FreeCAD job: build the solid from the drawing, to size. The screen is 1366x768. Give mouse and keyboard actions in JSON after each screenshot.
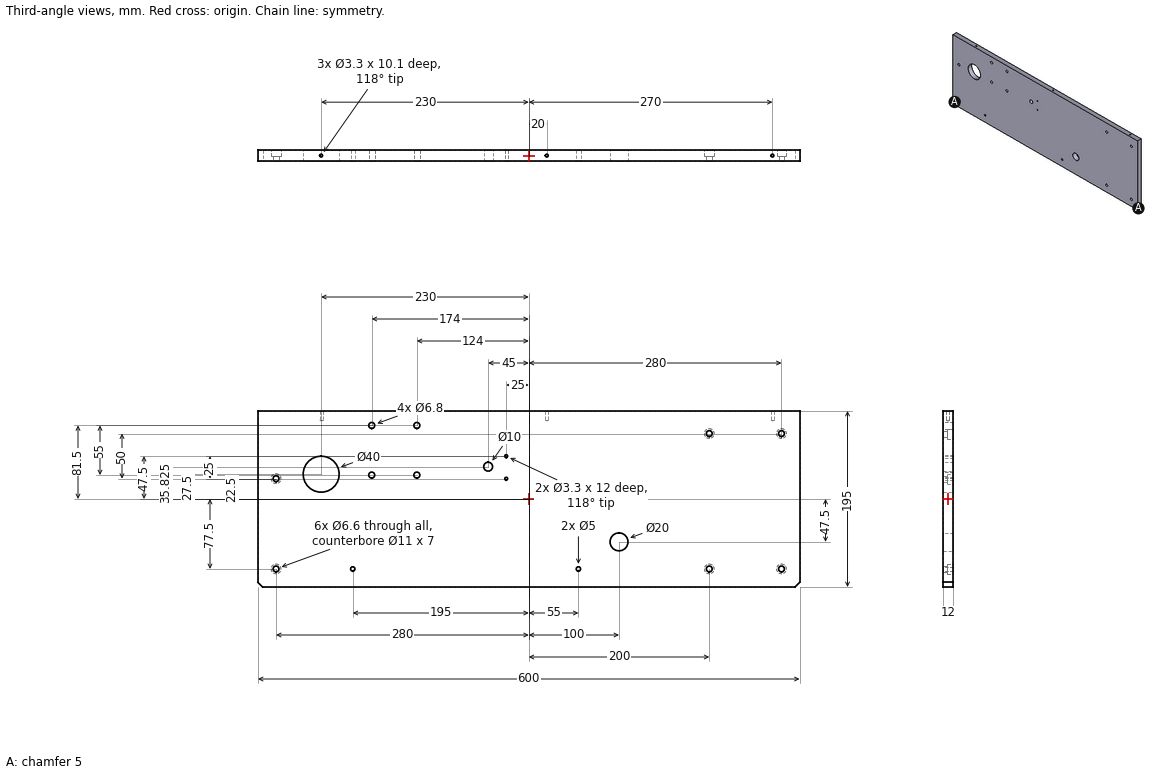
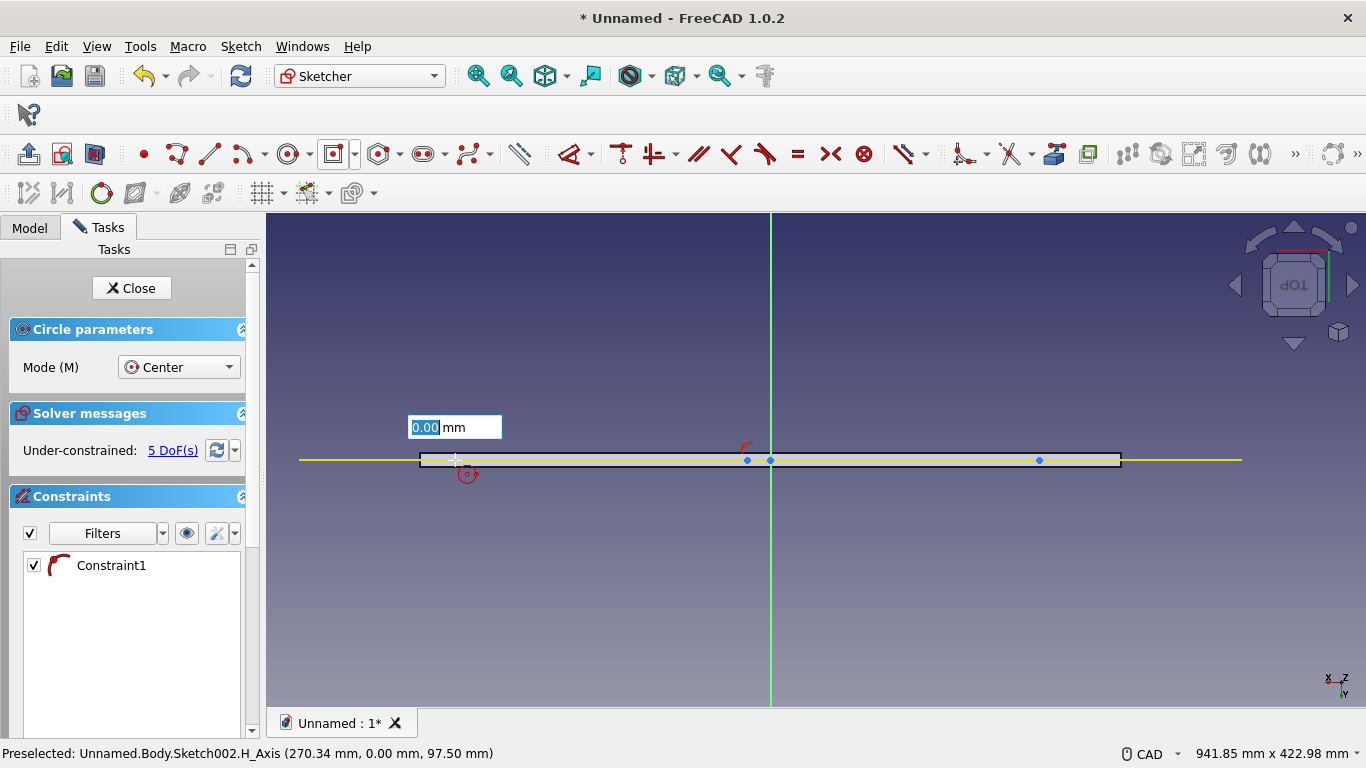
{"action": "scroll", "coordinate": [455, 462], "scroll_direction": "up", "scroll_amount": 11}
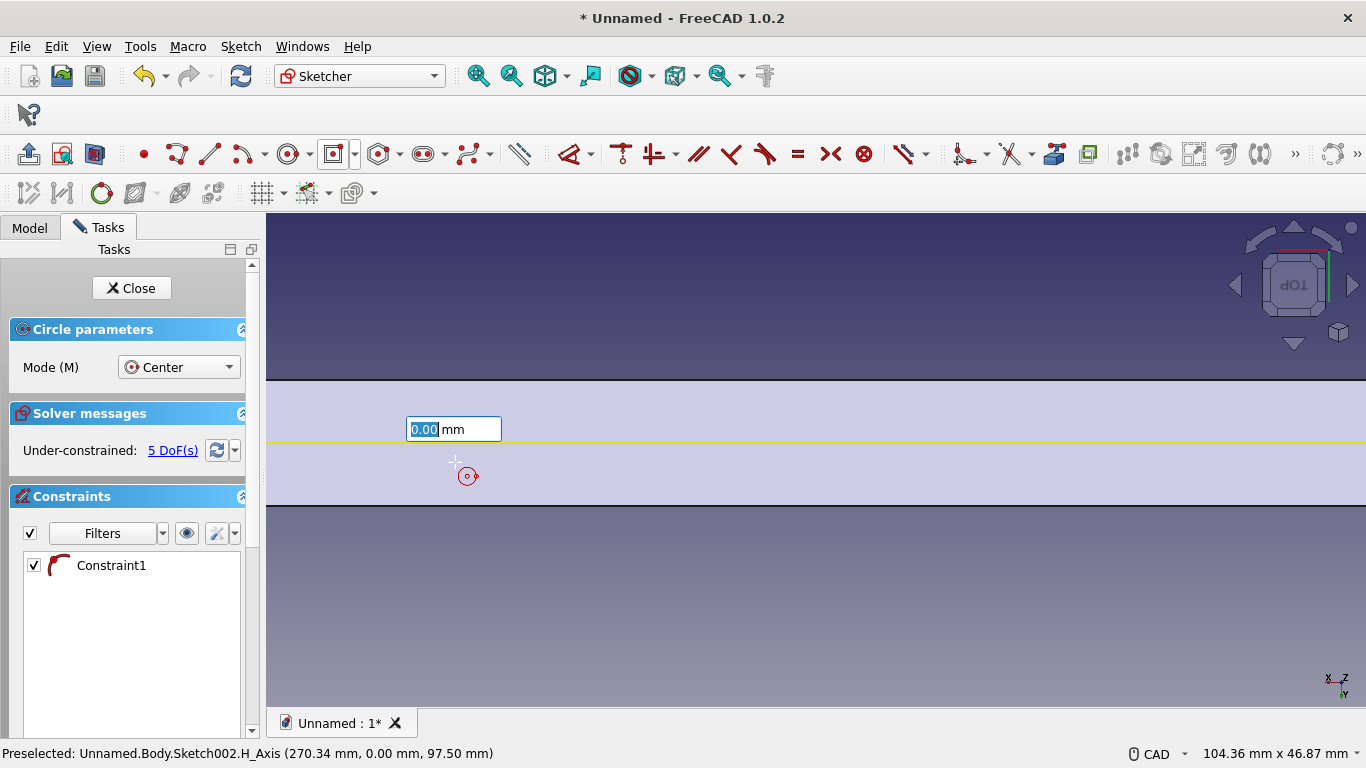
{"action": "left_click", "coordinate": [451, 459]}
{"action": "key", "text": "Escape"}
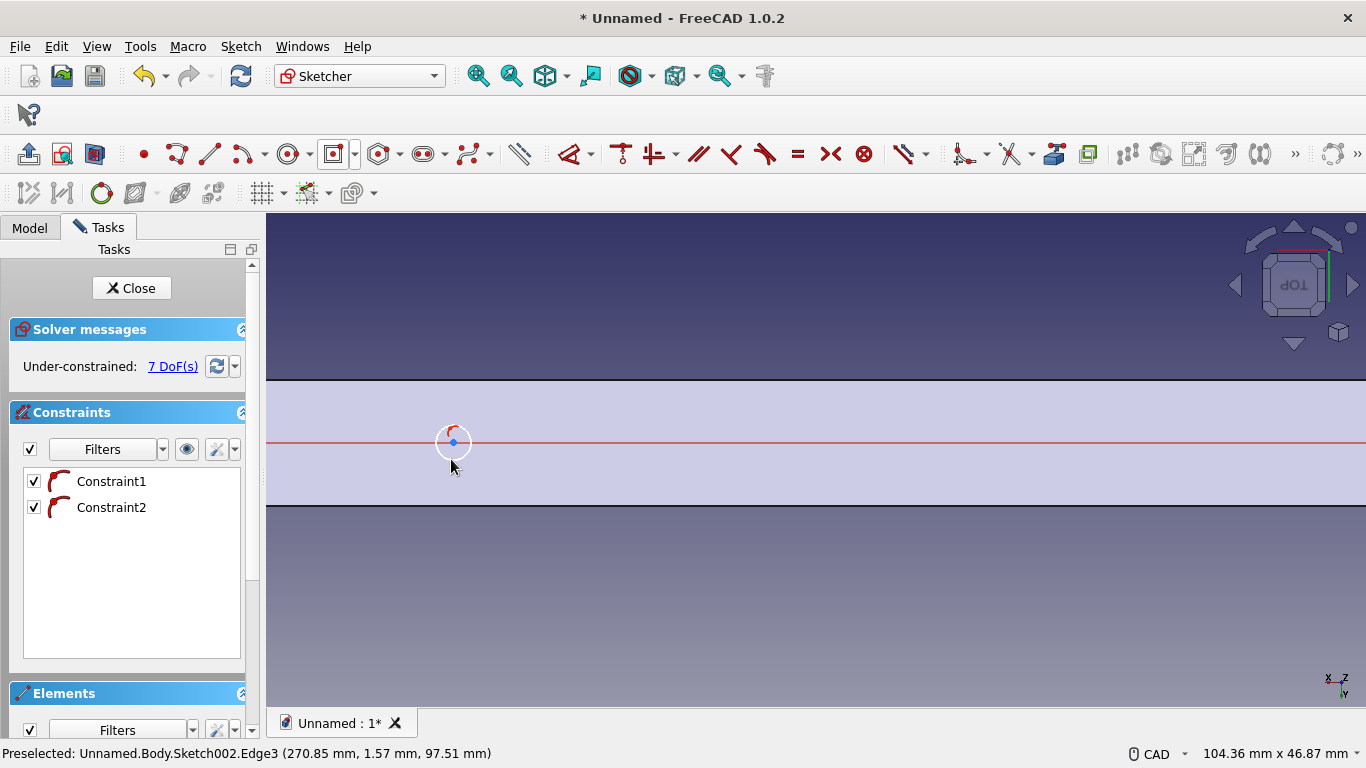
{"action": "scroll", "coordinate": [455, 462], "scroll_direction": "down", "scroll_amount": 11}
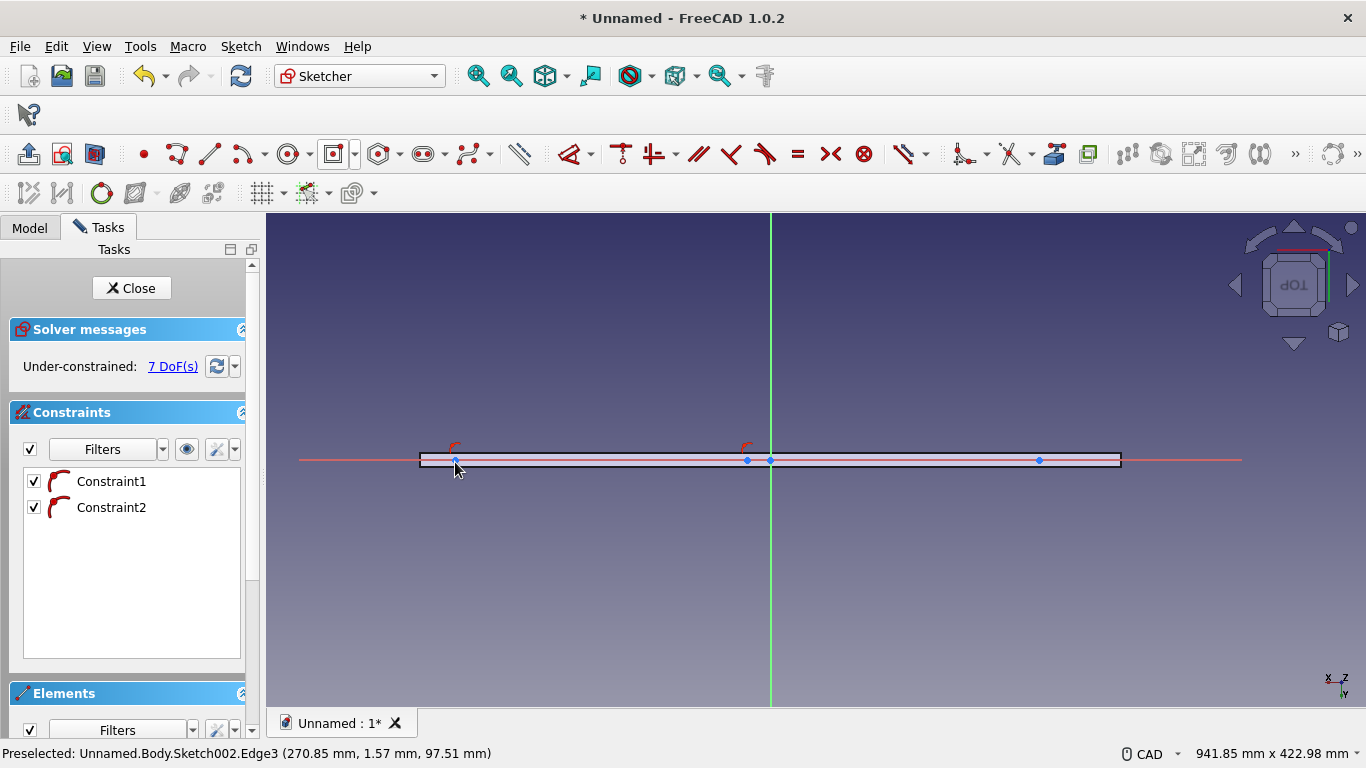
{"action": "scroll", "coordinate": [1040, 460], "scroll_direction": "up", "scroll_amount": 12}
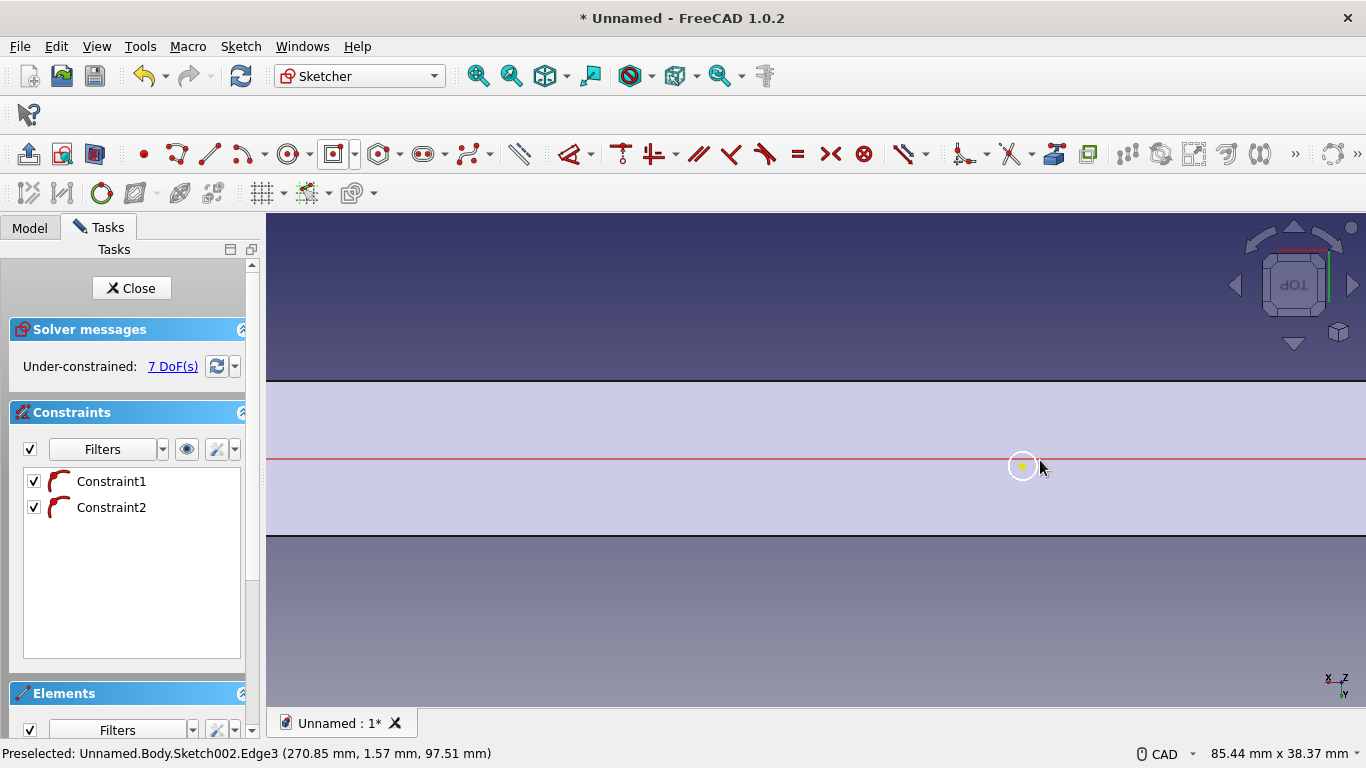
{"action": "left_click", "coordinate": [1033, 456]}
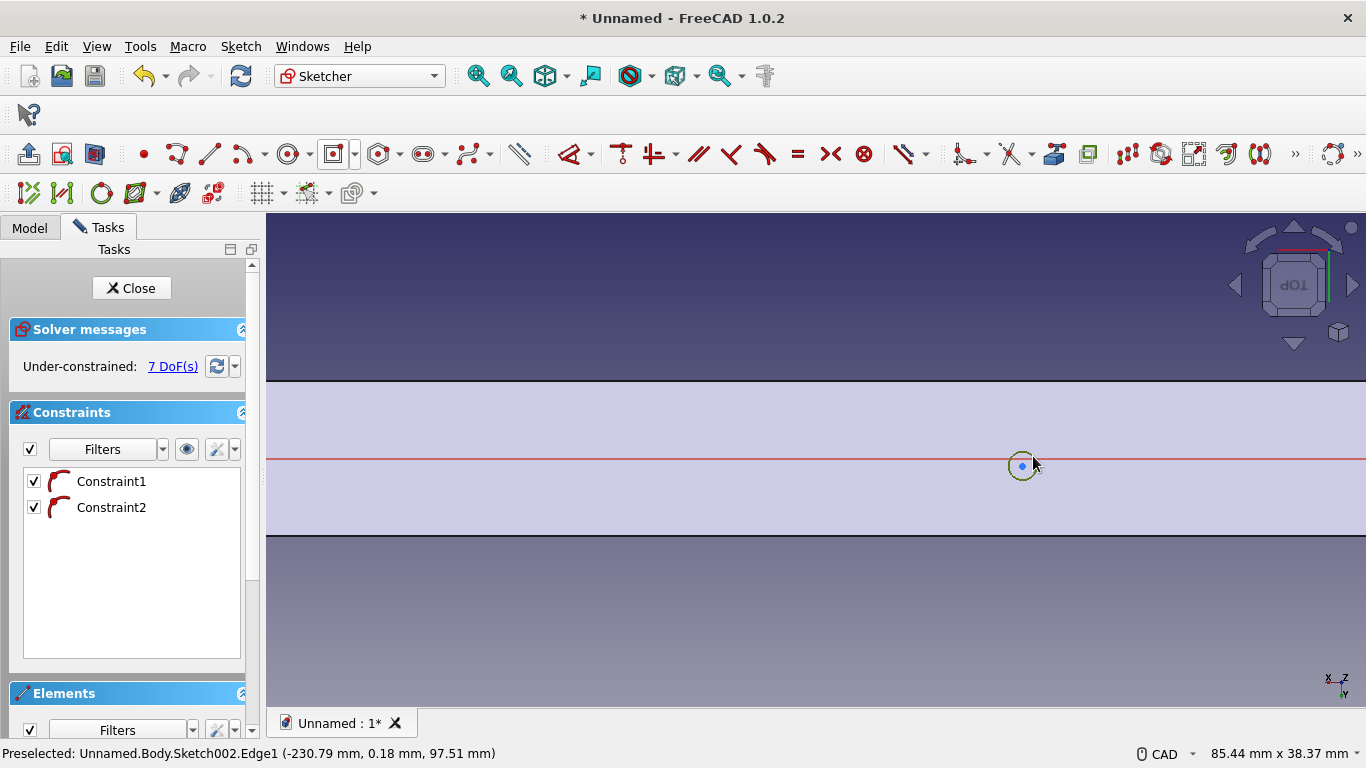
{"action": "scroll", "coordinate": [1041, 460], "scroll_direction": "down", "scroll_amount": 12}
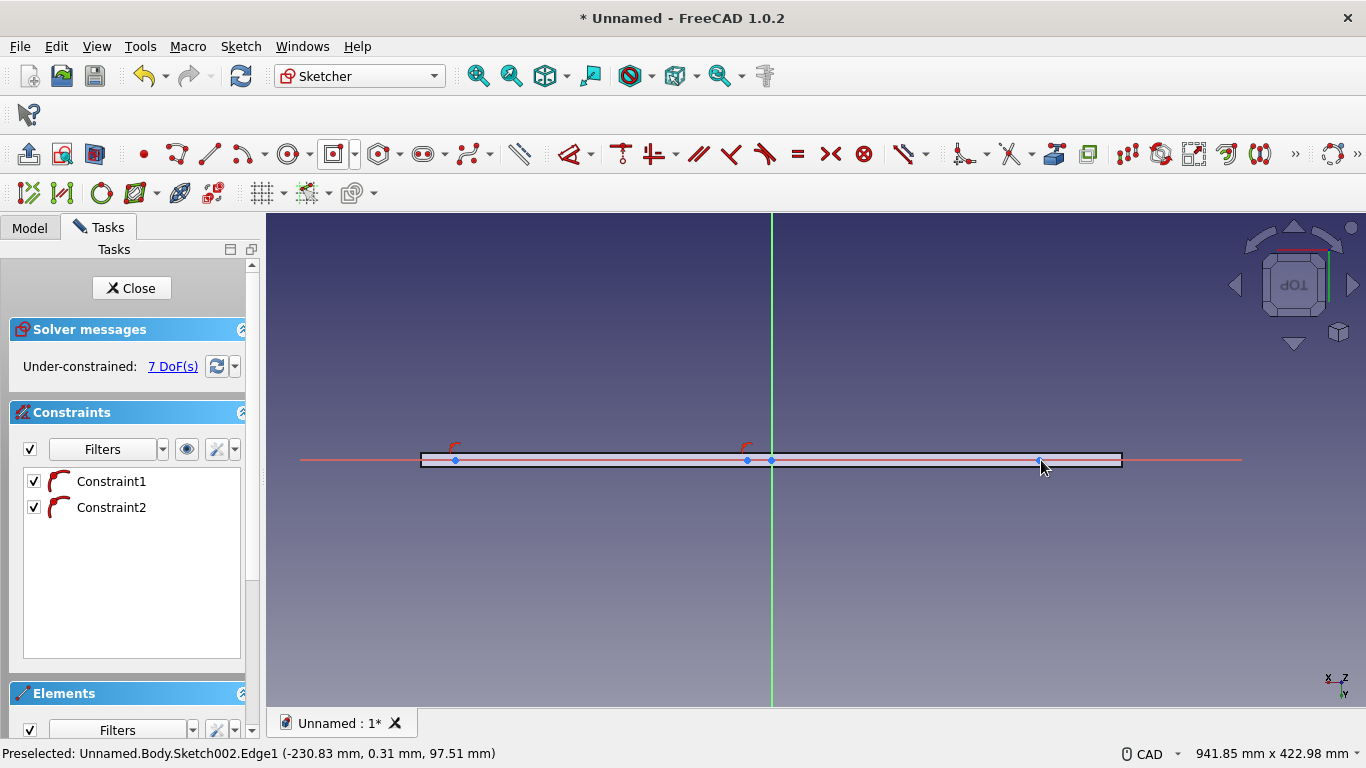
{"action": "scroll", "coordinate": [749, 459], "scroll_direction": "up", "scroll_amount": 12}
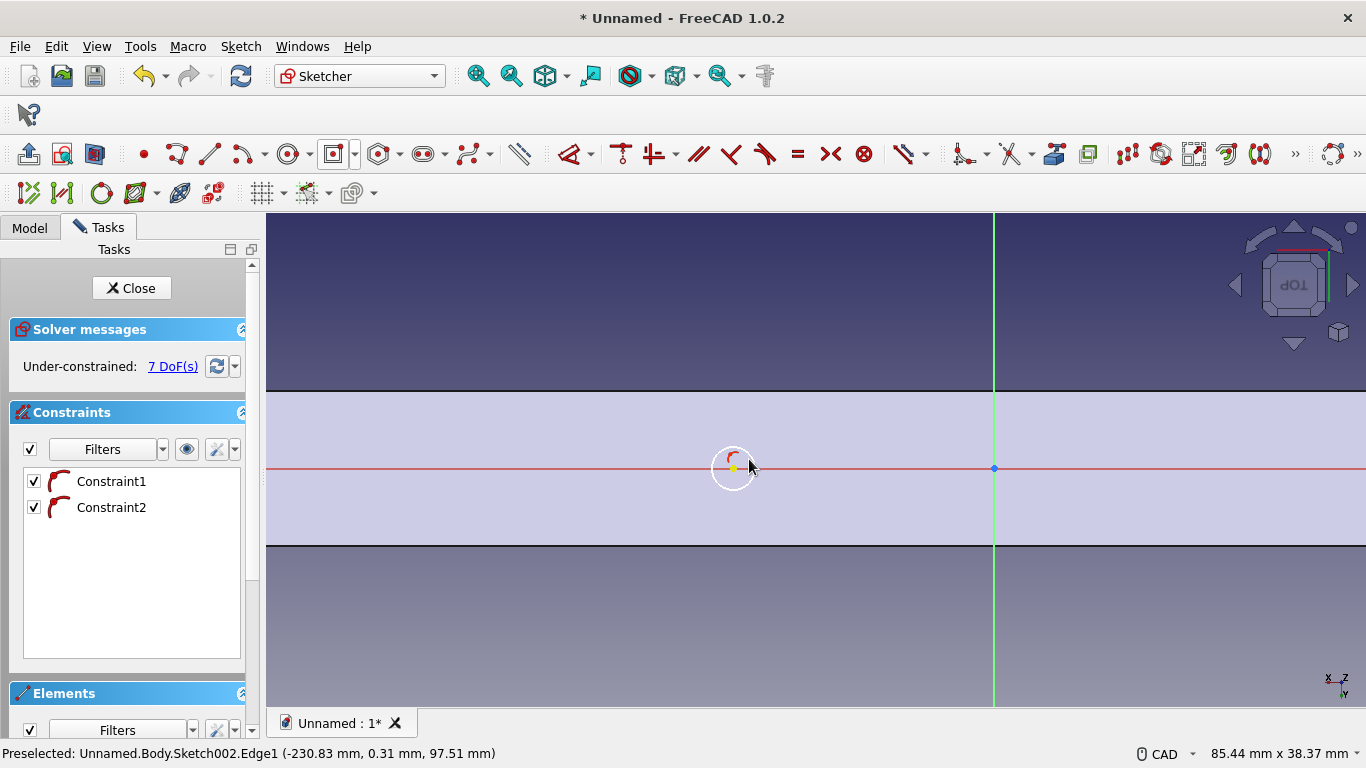
{"action": "left_click", "coordinate": [748, 453]}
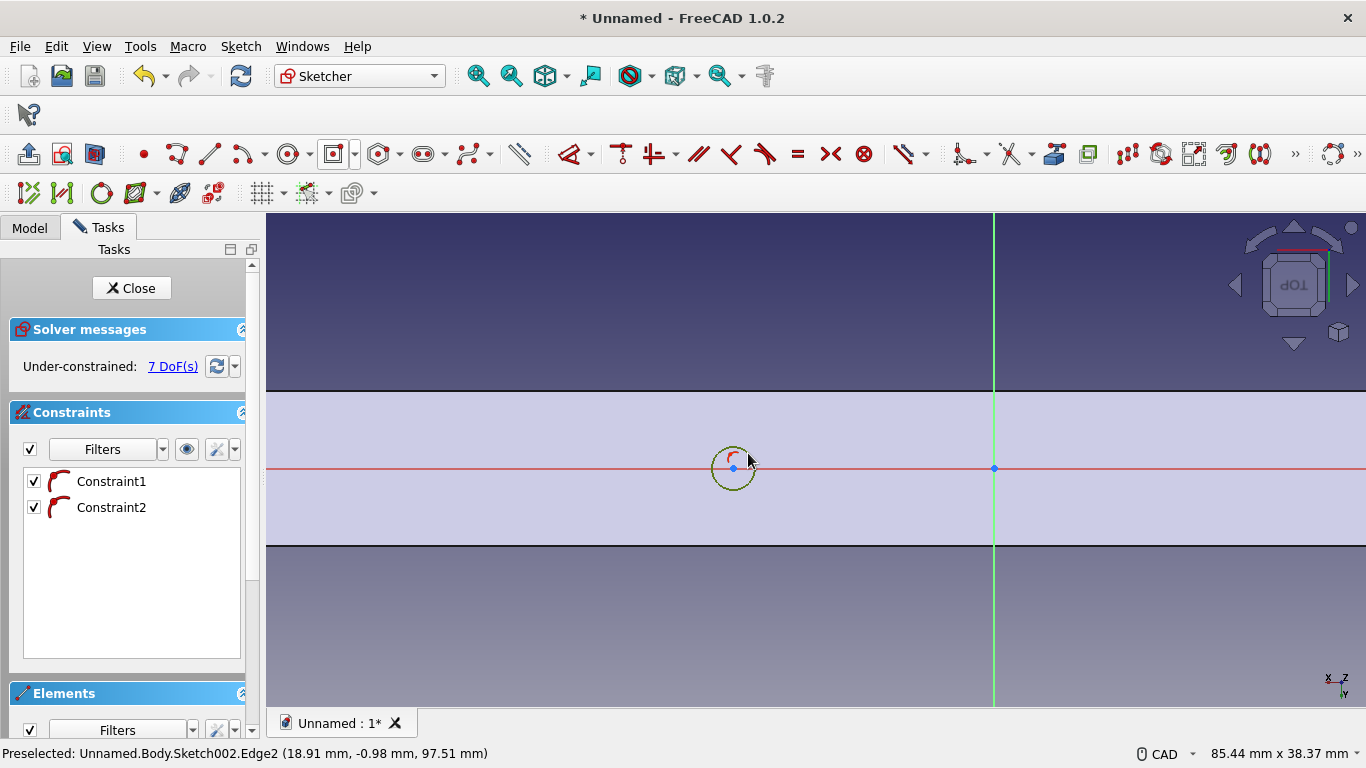
{"action": "scroll", "coordinate": [749, 459], "scroll_direction": "down", "scroll_amount": 12}